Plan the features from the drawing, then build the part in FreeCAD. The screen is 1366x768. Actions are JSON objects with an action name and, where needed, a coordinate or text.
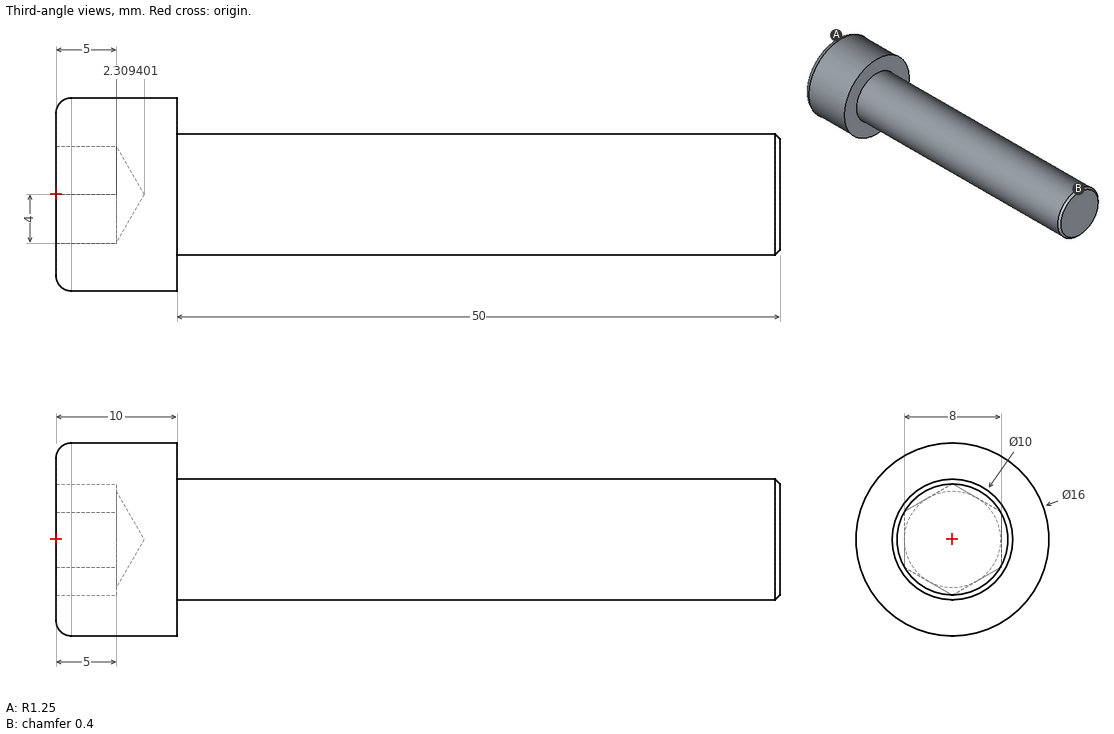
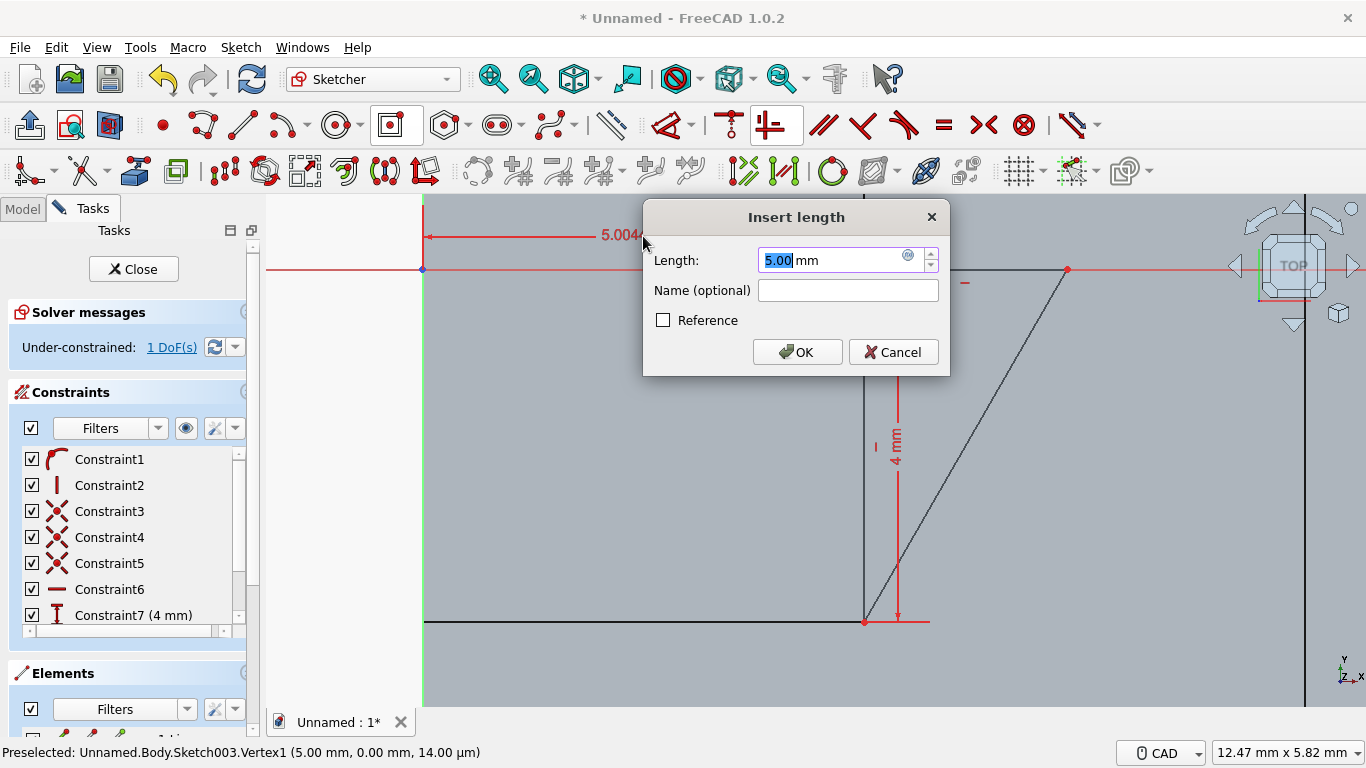
{"action": "type", "text": "5"}
{"action": "key", "text": "Return"}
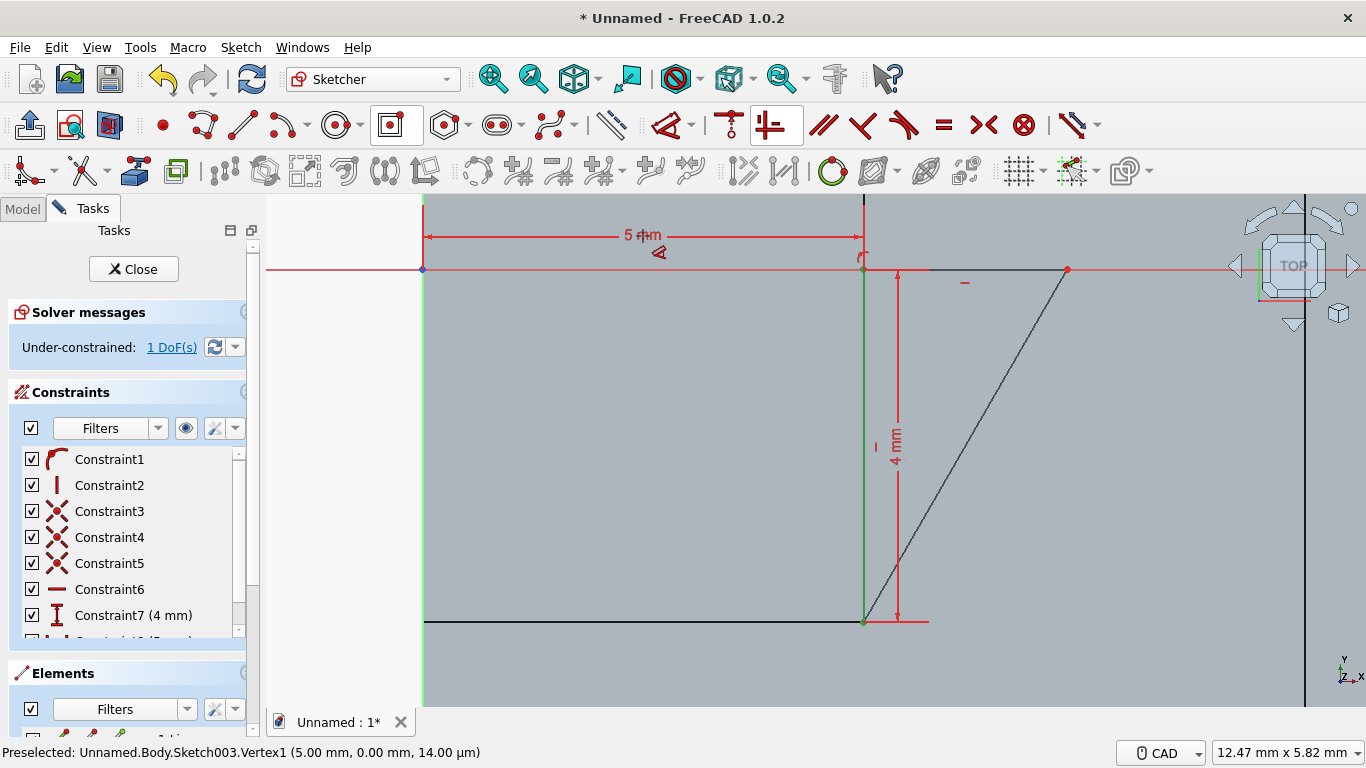
{"action": "left_click", "coordinate": [1006, 270]}
{"action": "left_click", "coordinate": [965, 236]}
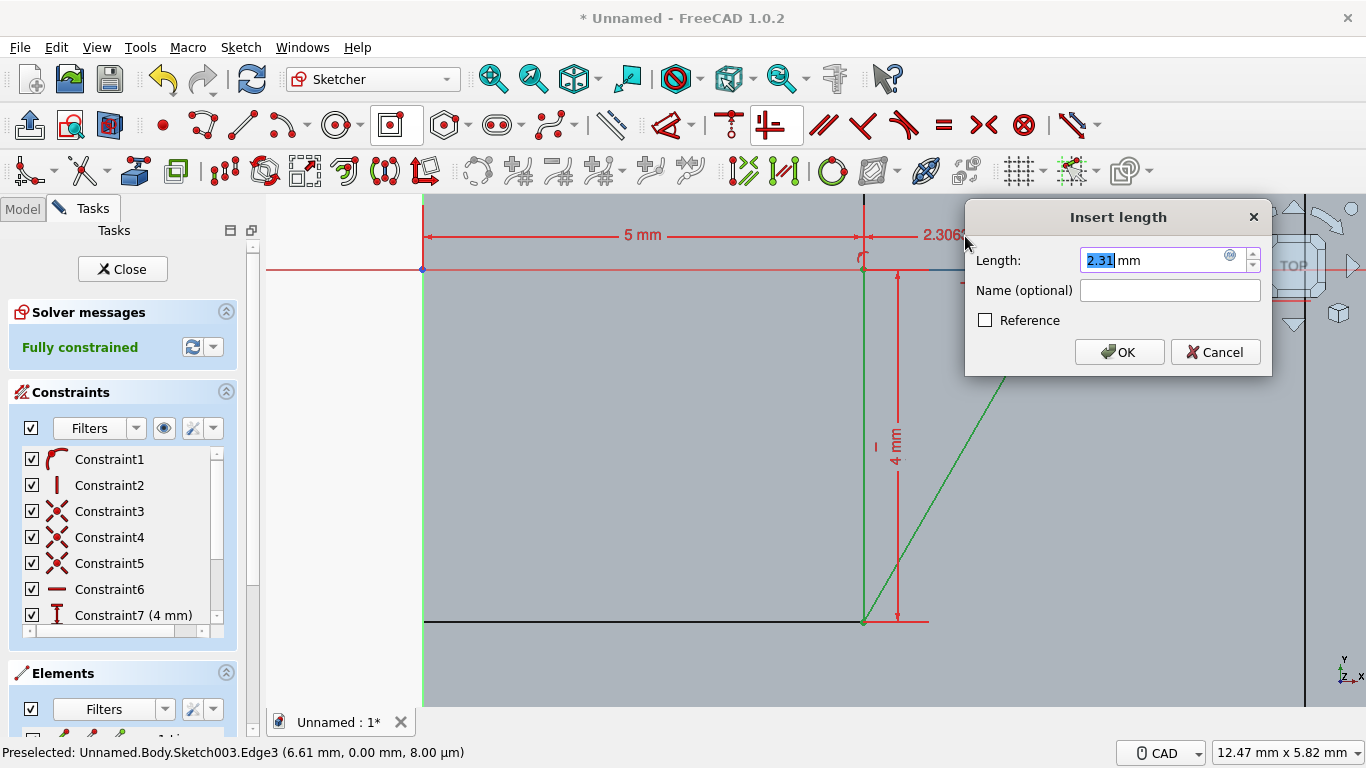
{"action": "type", "text": "2.309401"}
{"action": "key", "text": "Return"}
{"action": "key", "text": "Escape"}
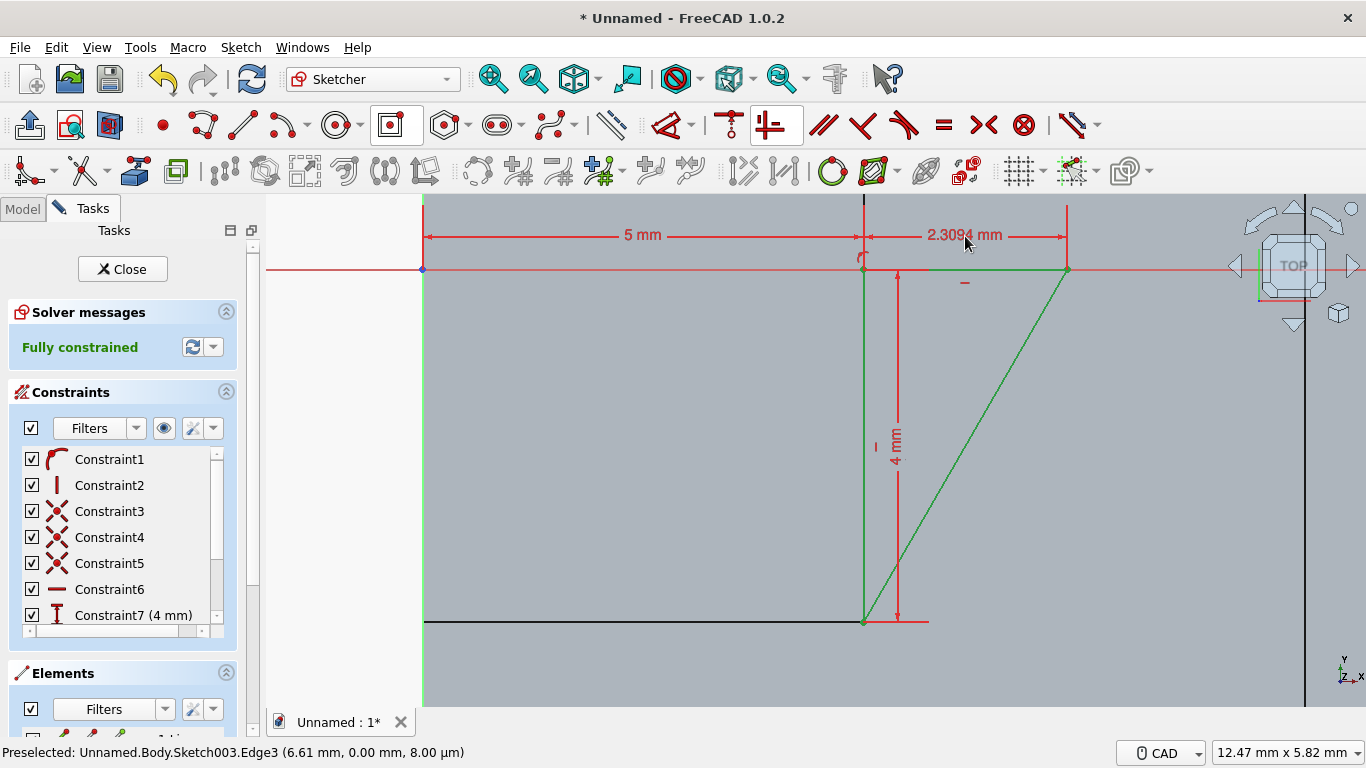
{"action": "left_click", "coordinate": [123, 269]}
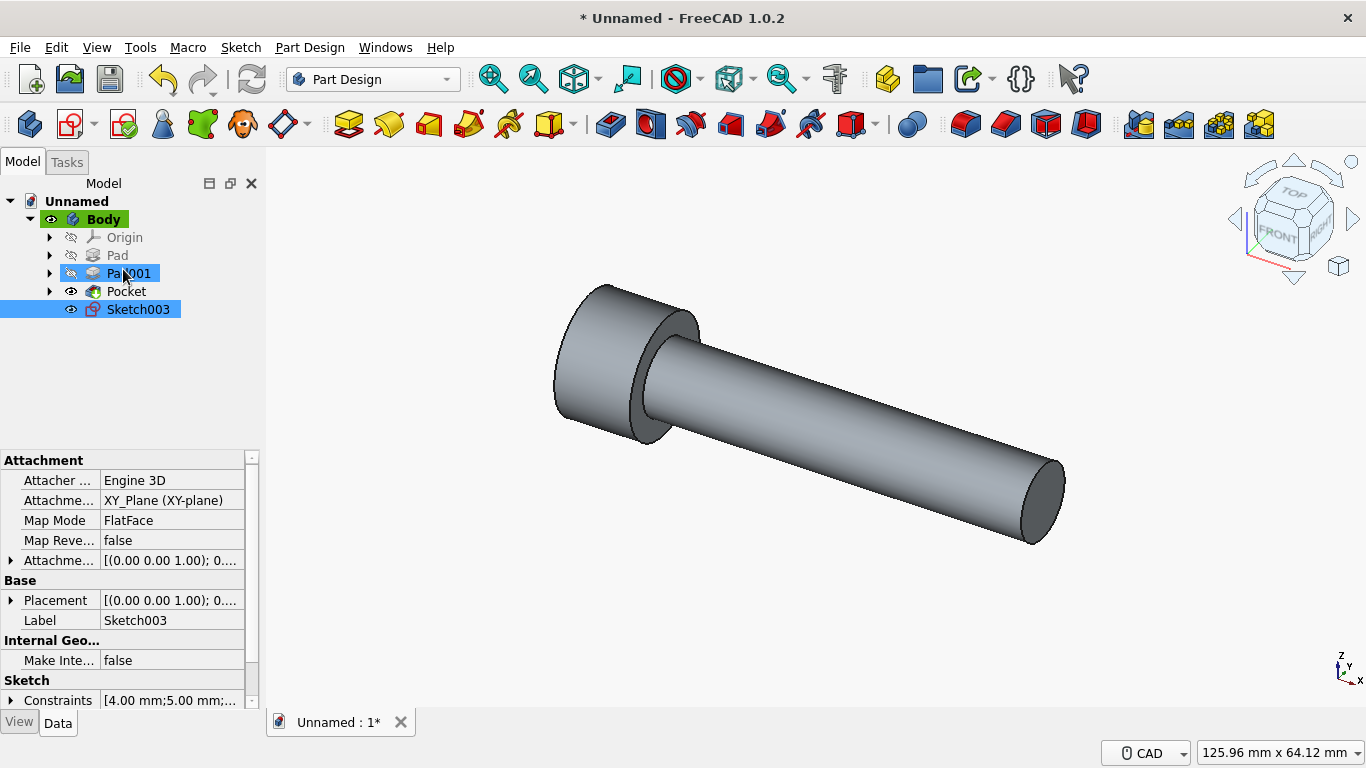
{"action": "left_click", "coordinate": [692, 124]}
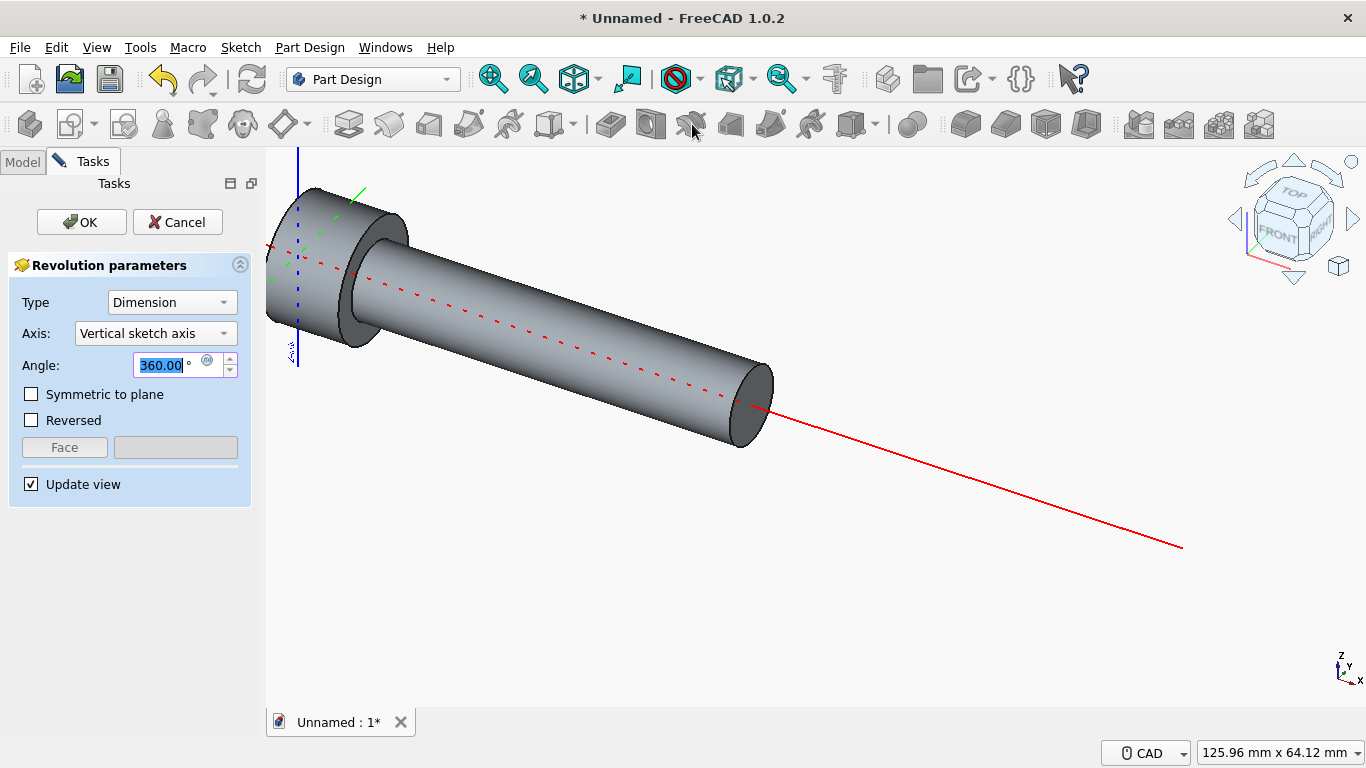
{"action": "left_click", "coordinate": [156, 334]}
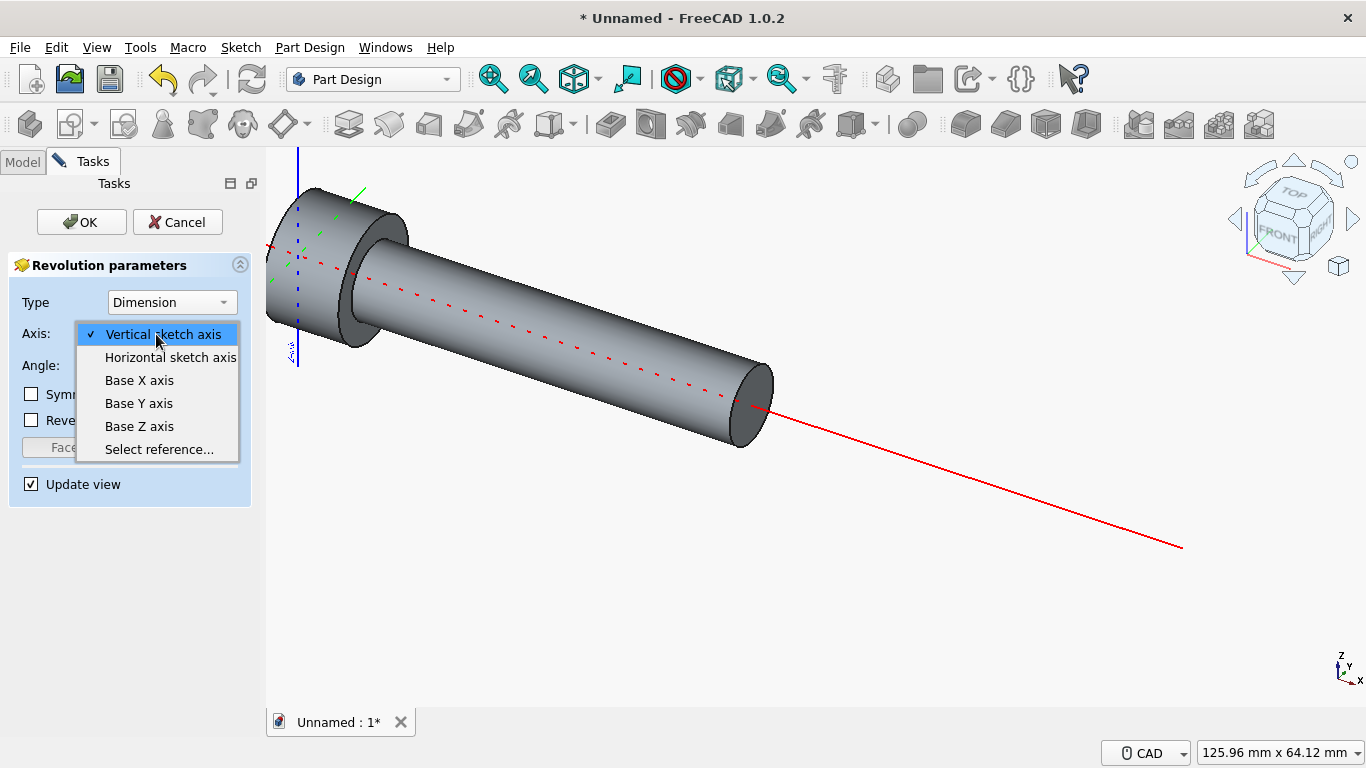
{"action": "left_click", "coordinate": [156, 358]}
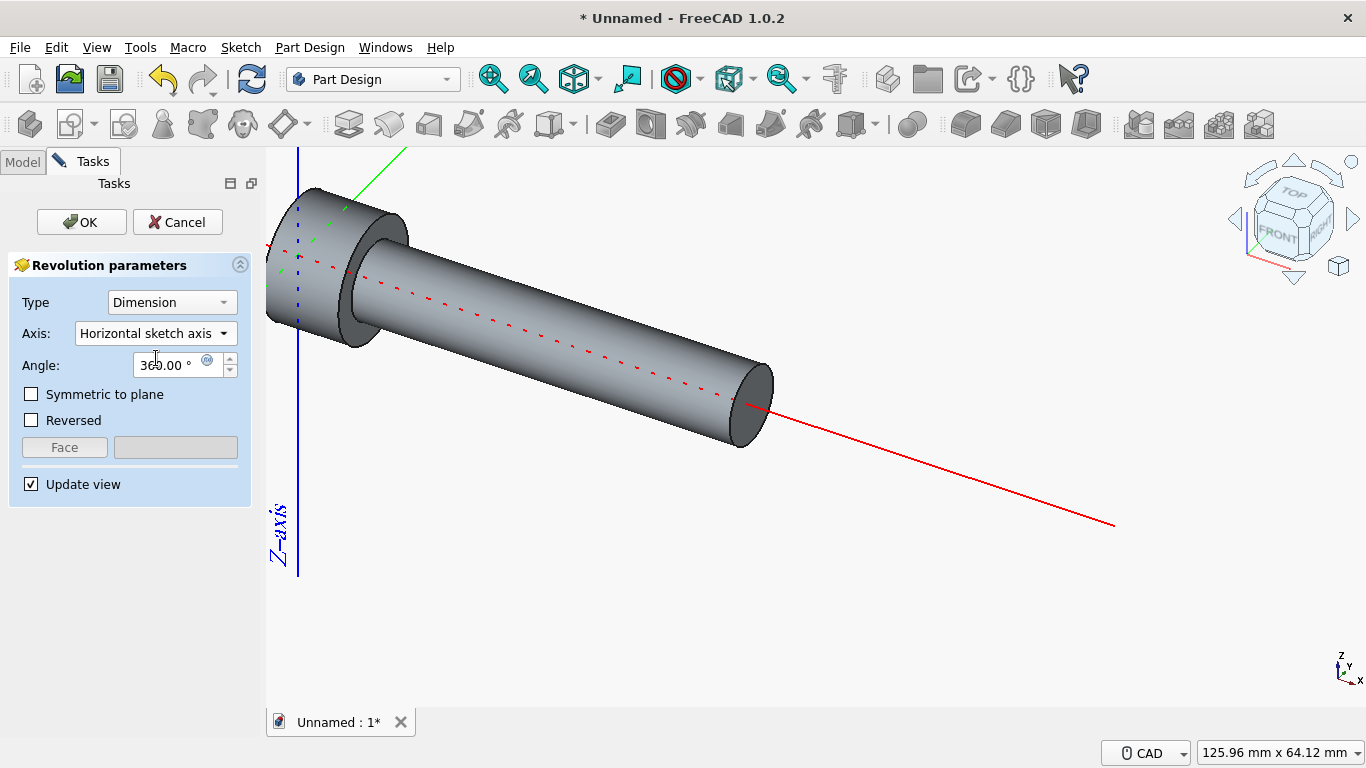
{"action": "left_click", "coordinate": [82, 222]}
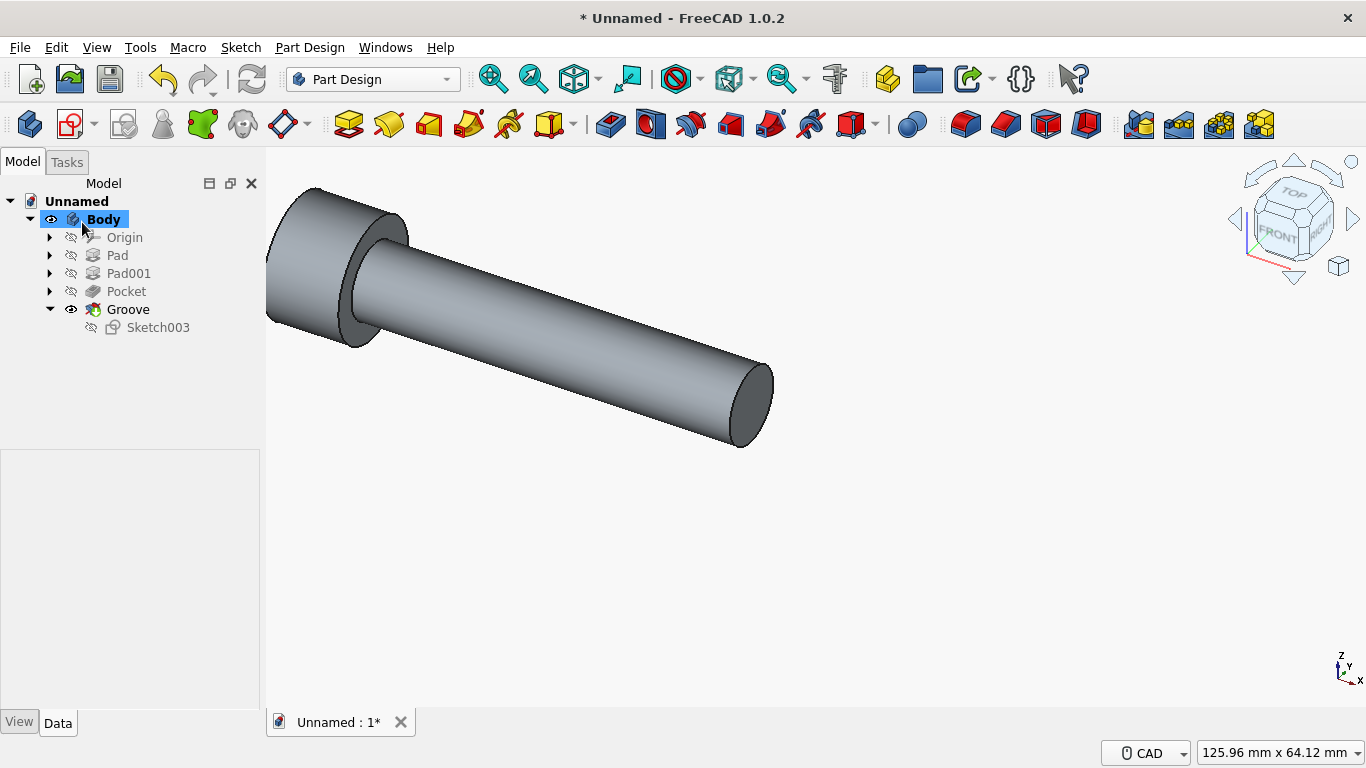
{"action": "key", "text": "v f"}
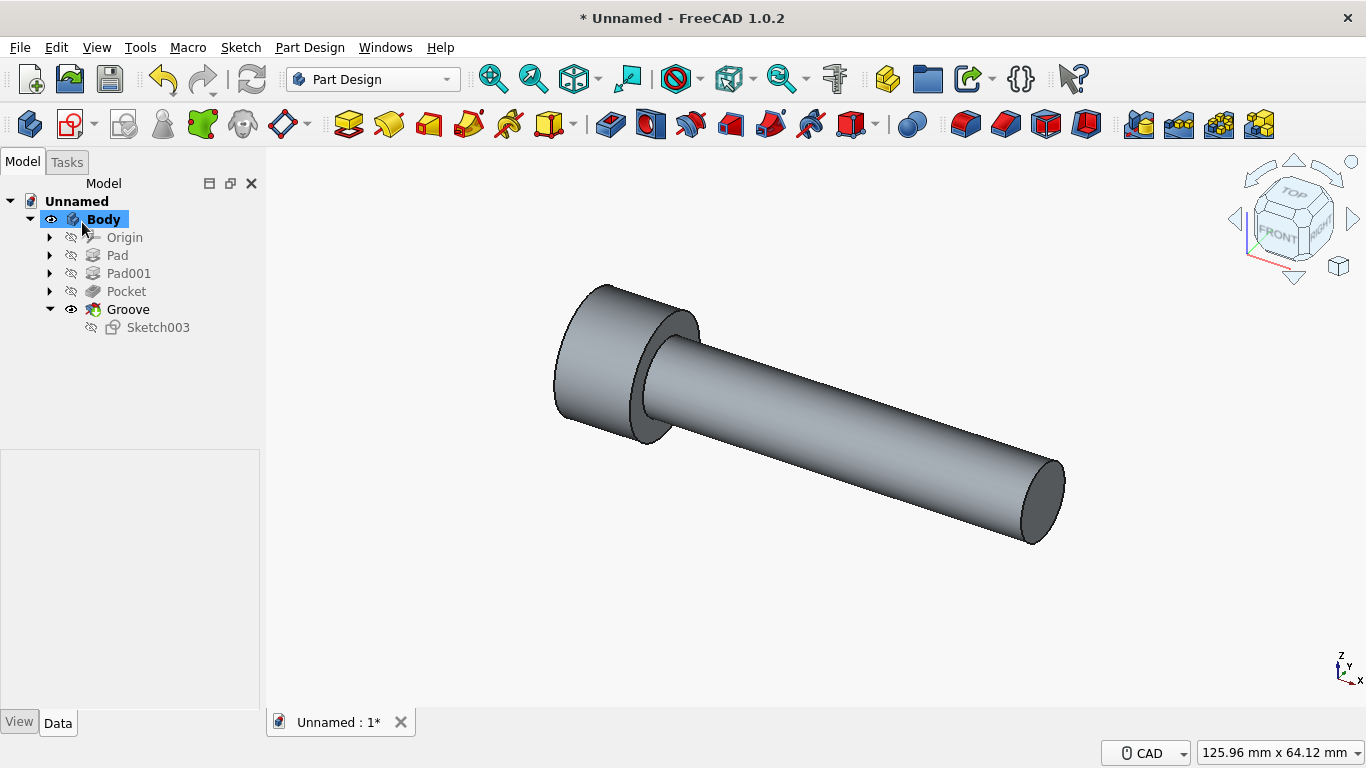
{"action": "left_click", "coordinate": [578, 307]}